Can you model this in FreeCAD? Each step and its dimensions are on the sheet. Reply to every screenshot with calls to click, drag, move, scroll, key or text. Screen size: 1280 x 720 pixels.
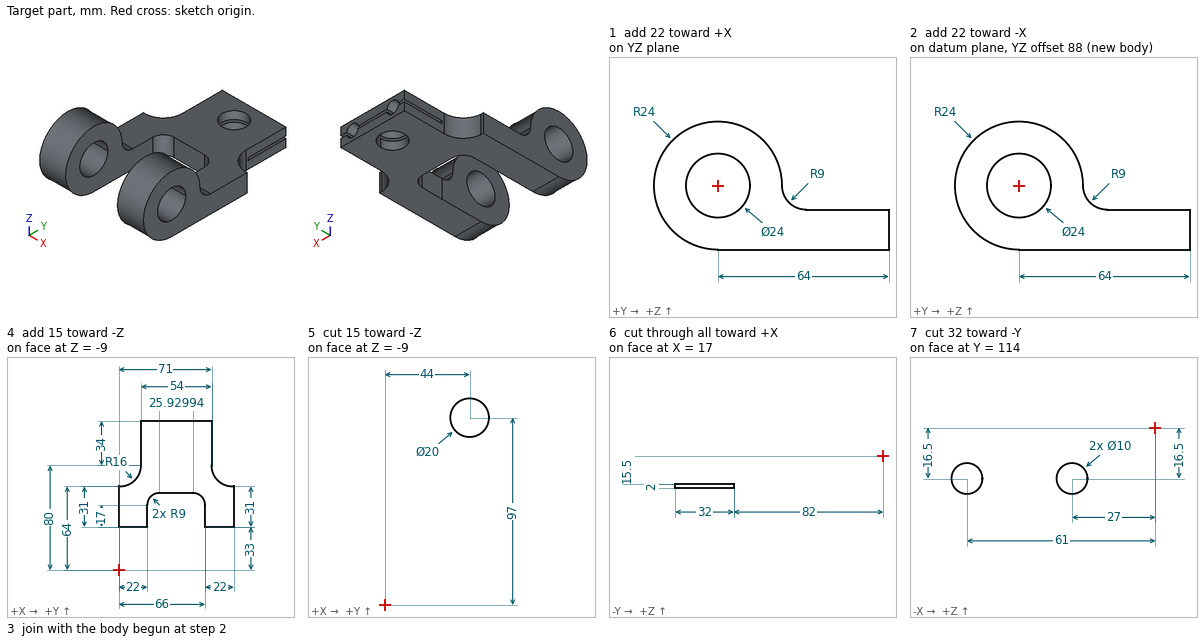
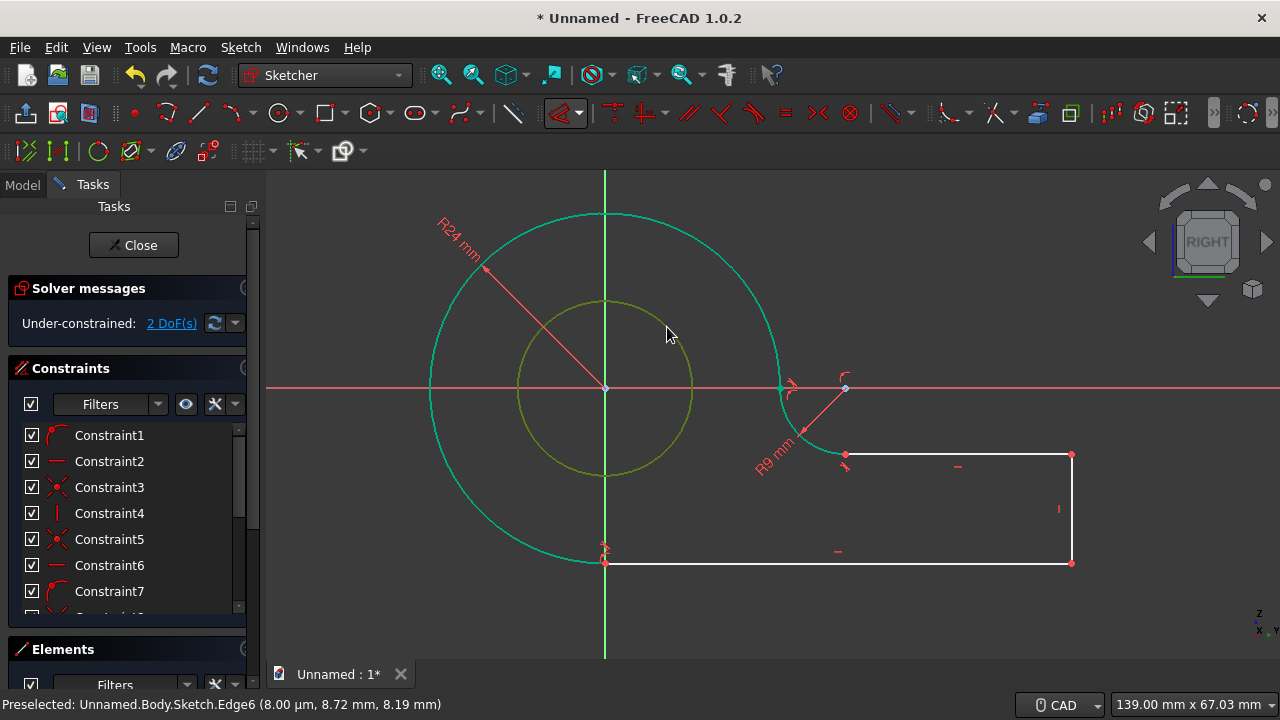
key(k)
key(o)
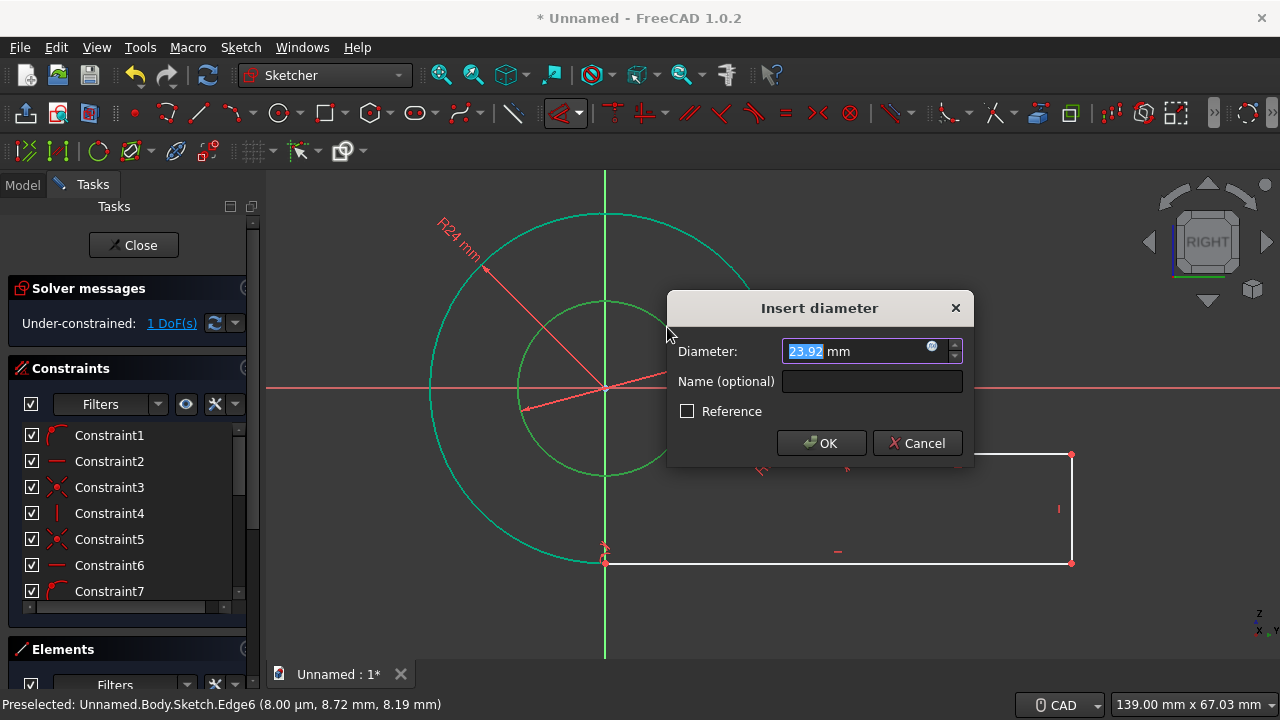
text(24)
key(Return)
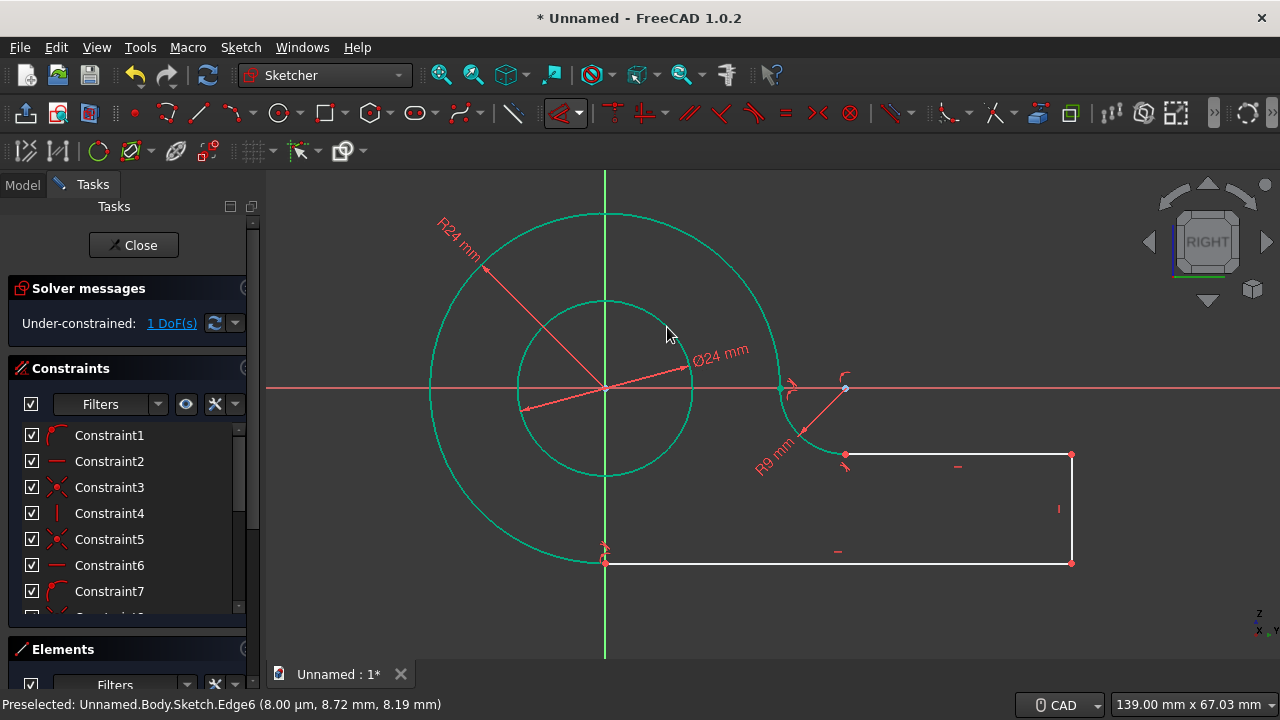
click(745, 564)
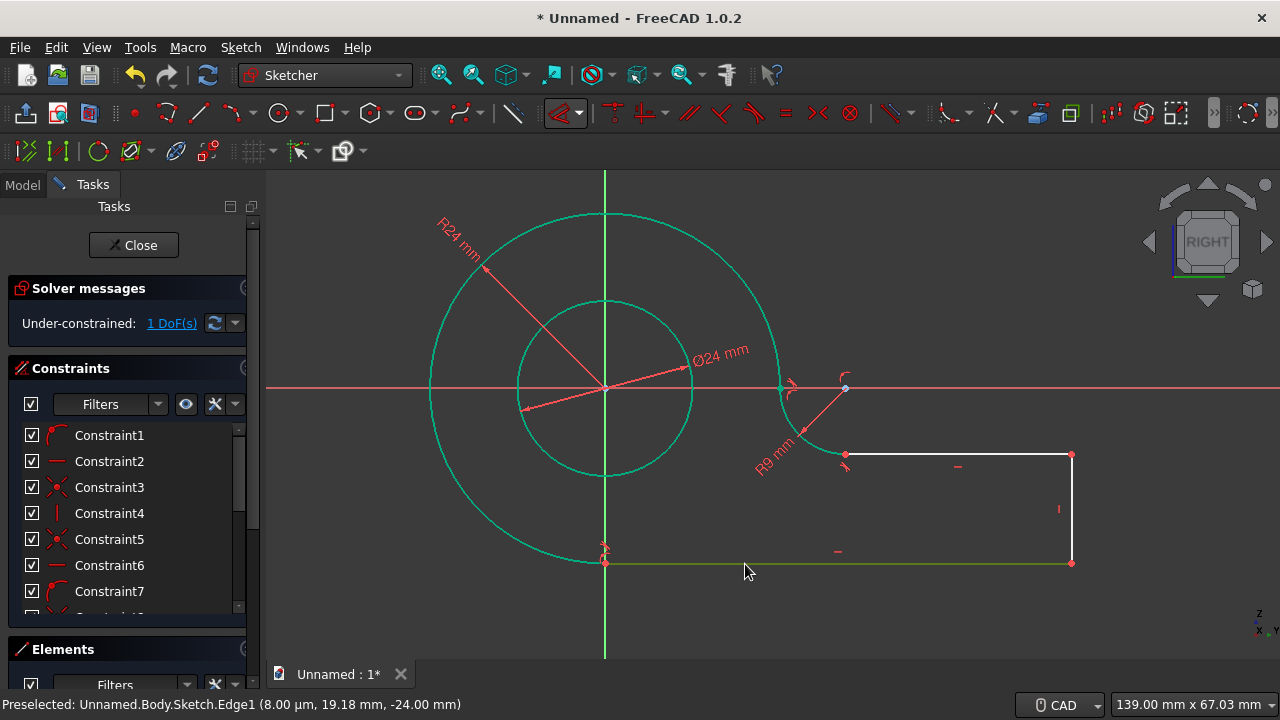
click(582, 114)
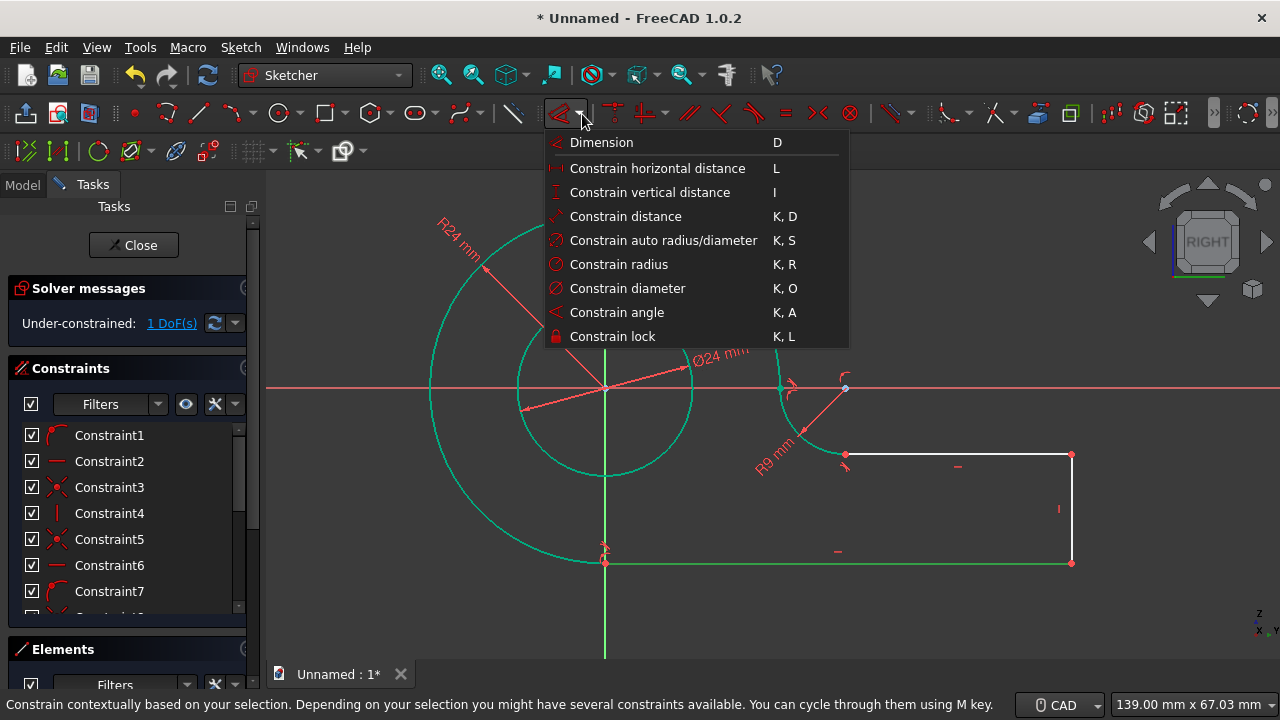
click(697, 168)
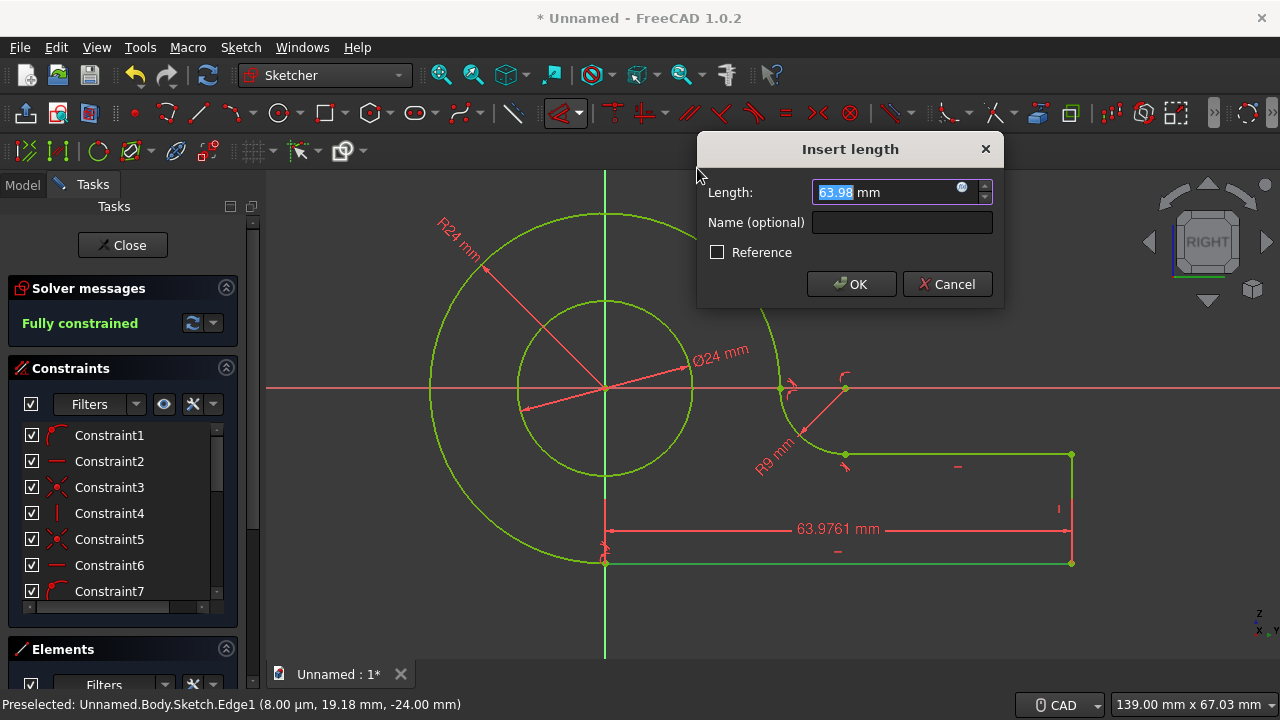
text(64)
key(Return)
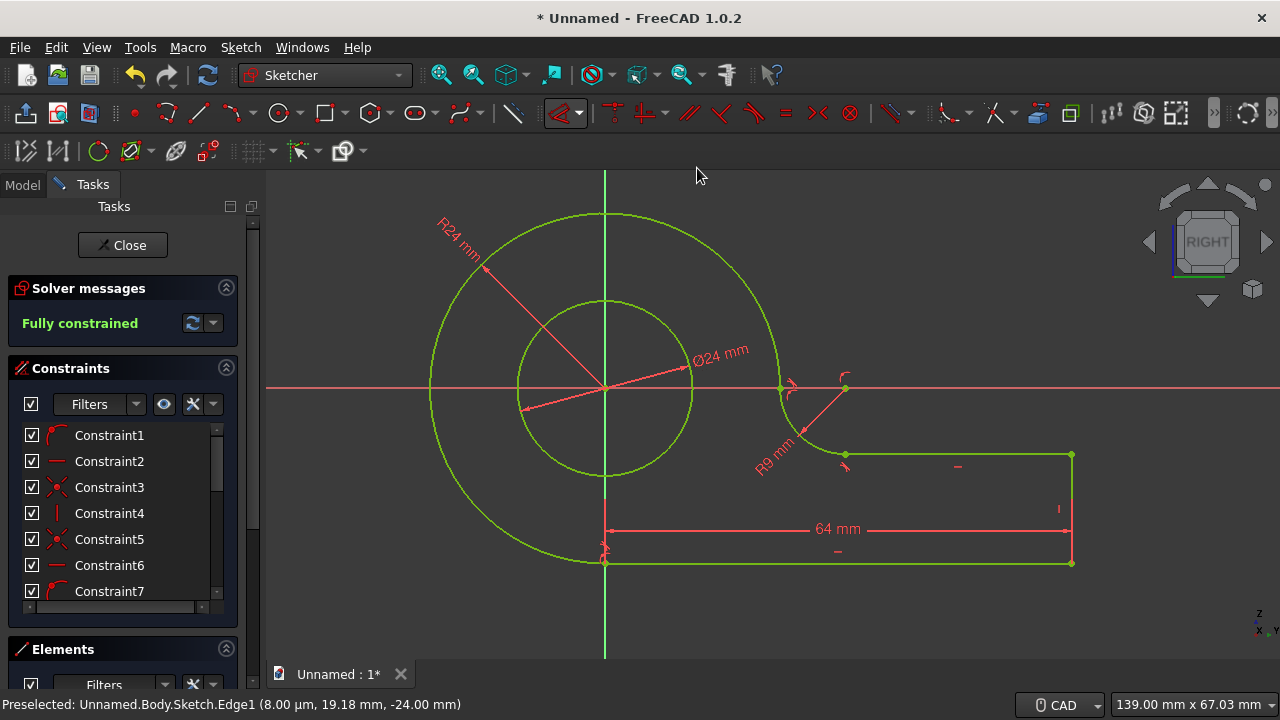
click(123, 245)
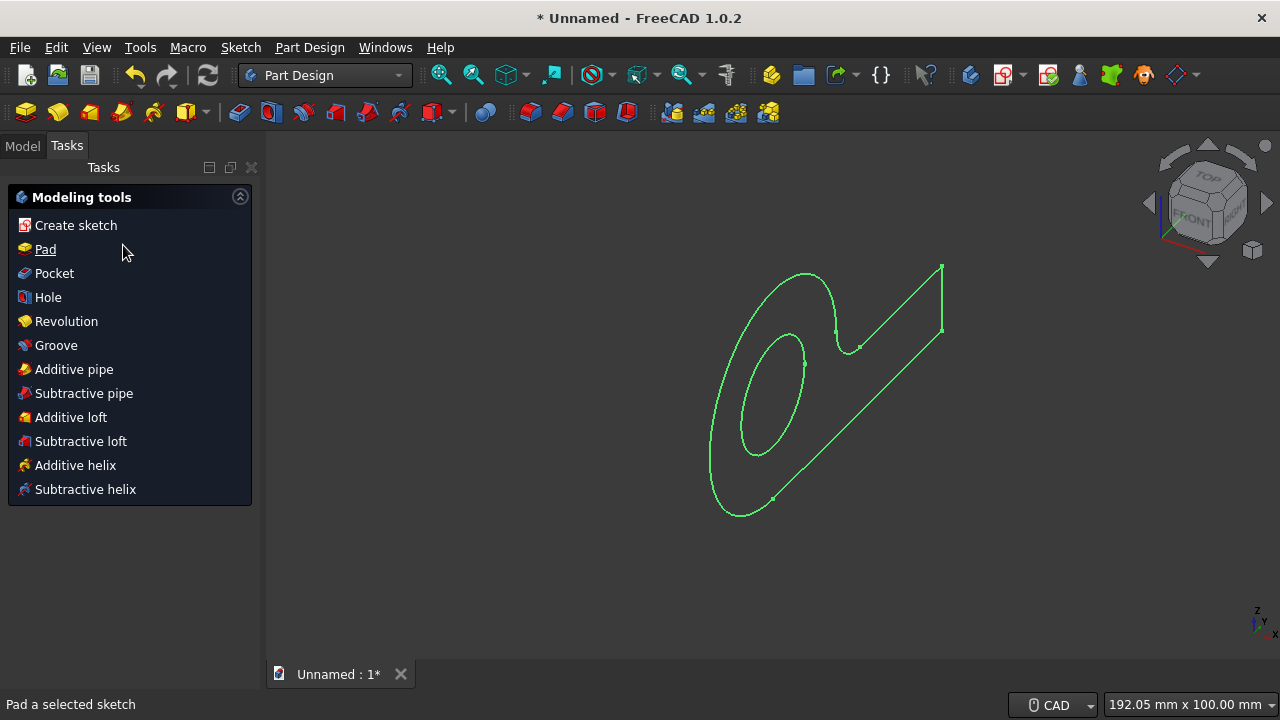
click(26, 112)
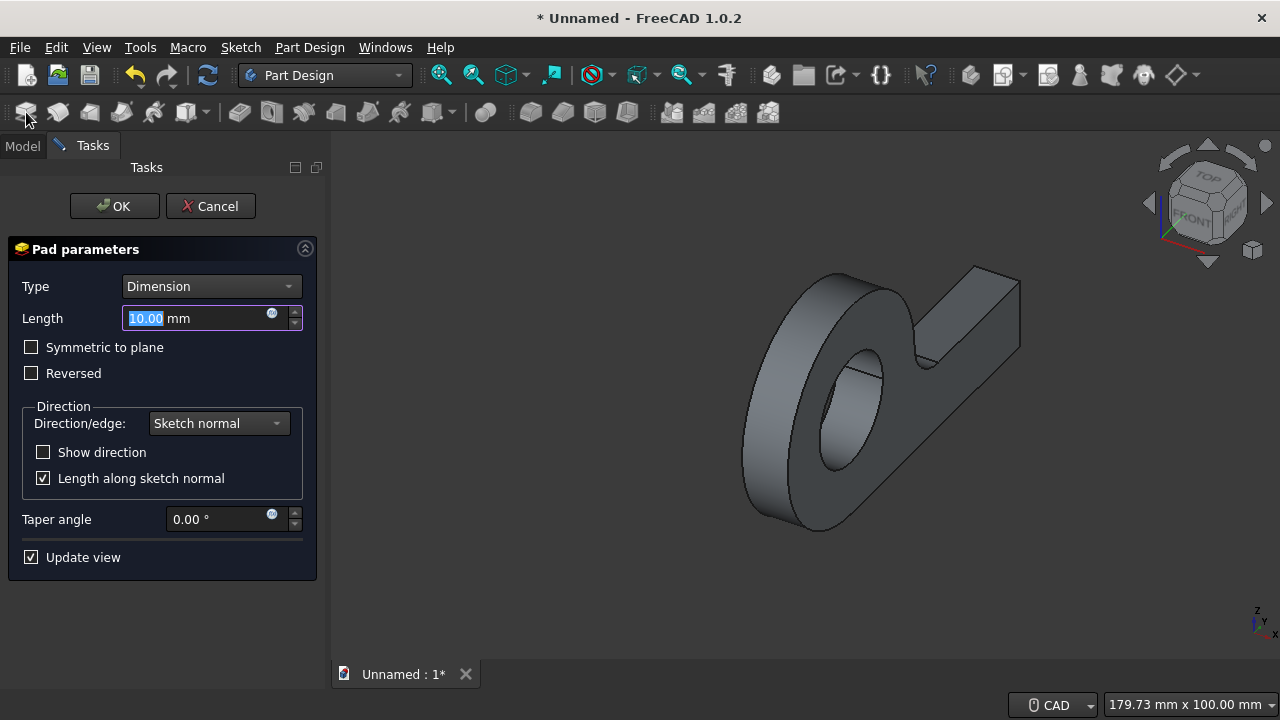
text(22)
key(Tab)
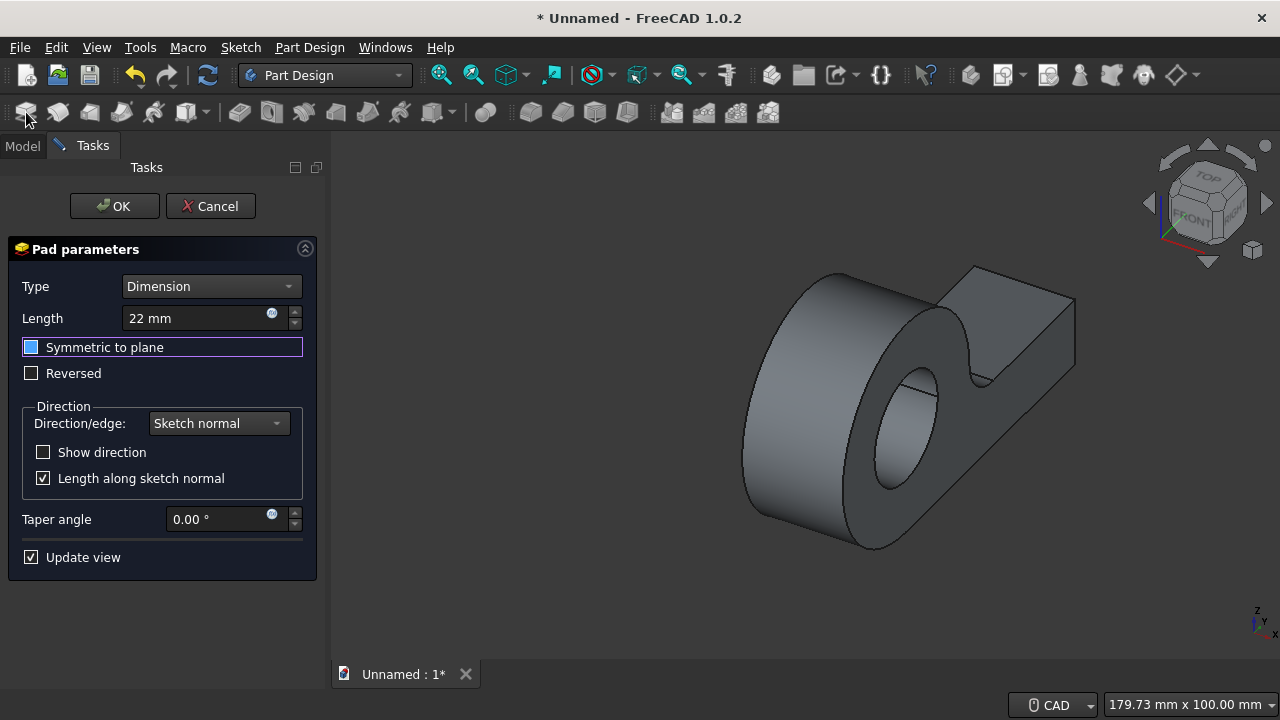
click(115, 206)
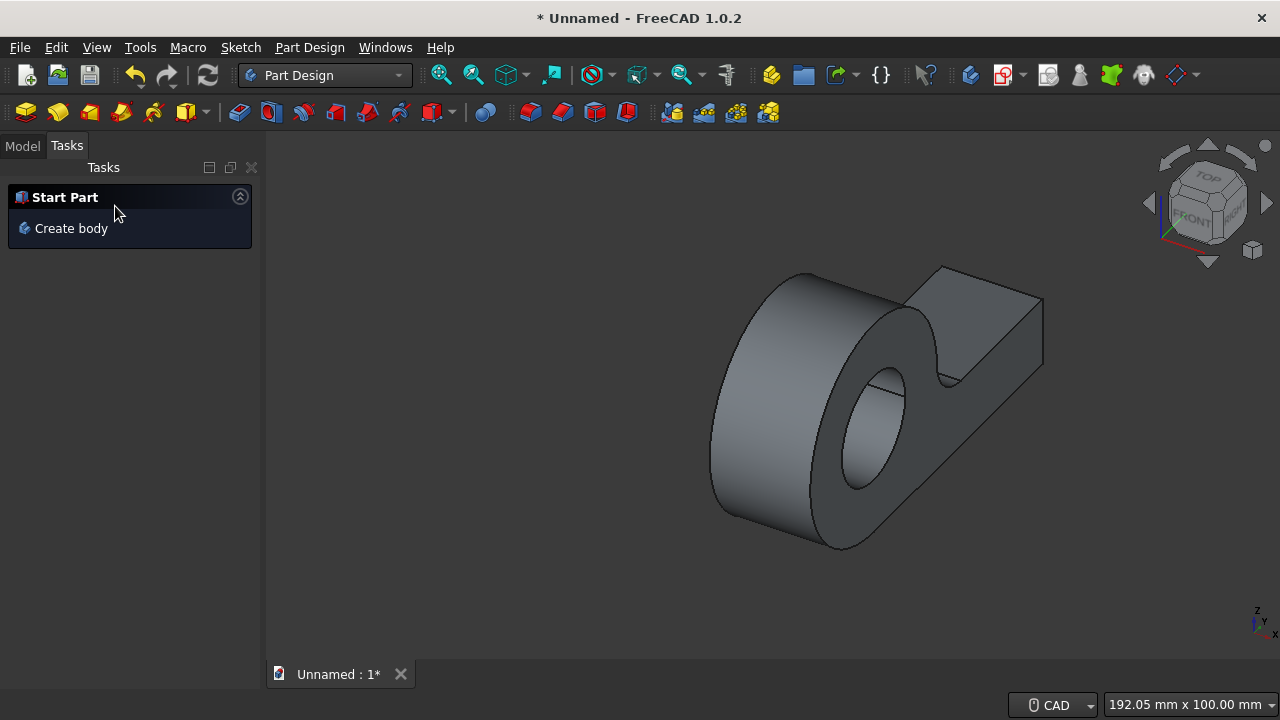
click(442, 76)